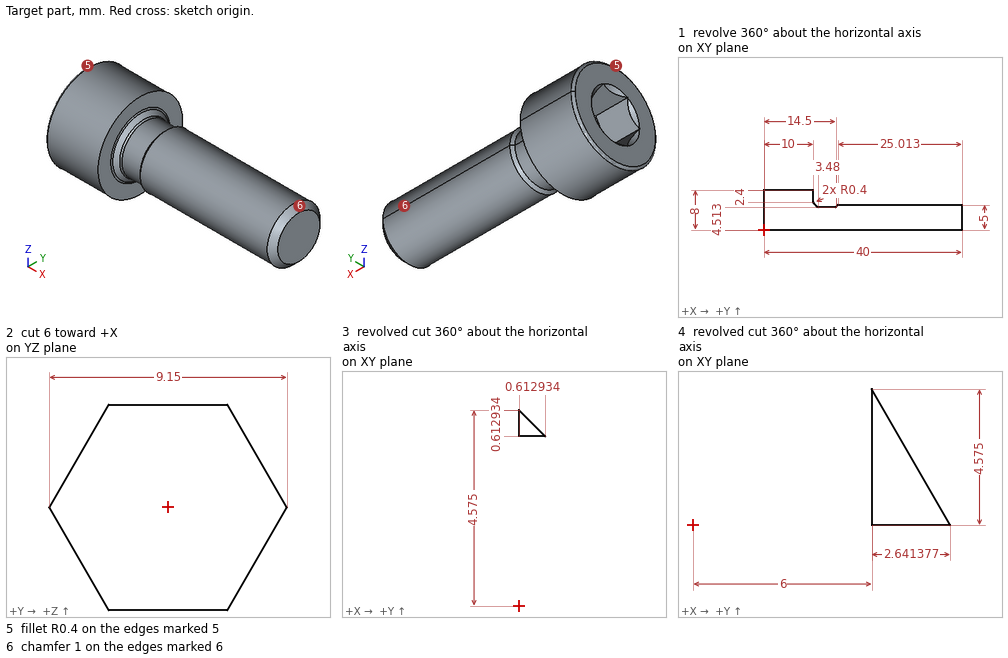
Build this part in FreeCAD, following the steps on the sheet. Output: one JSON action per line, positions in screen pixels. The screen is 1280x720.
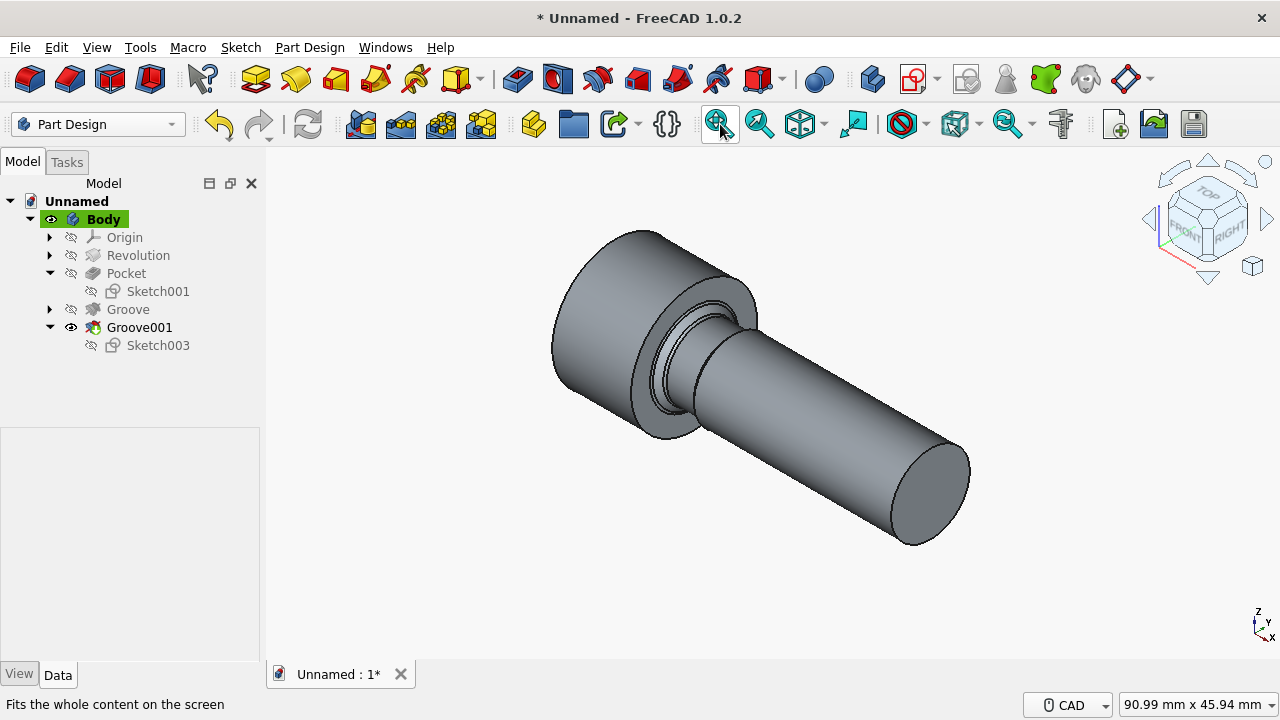
{"action": "key", "text": "2"}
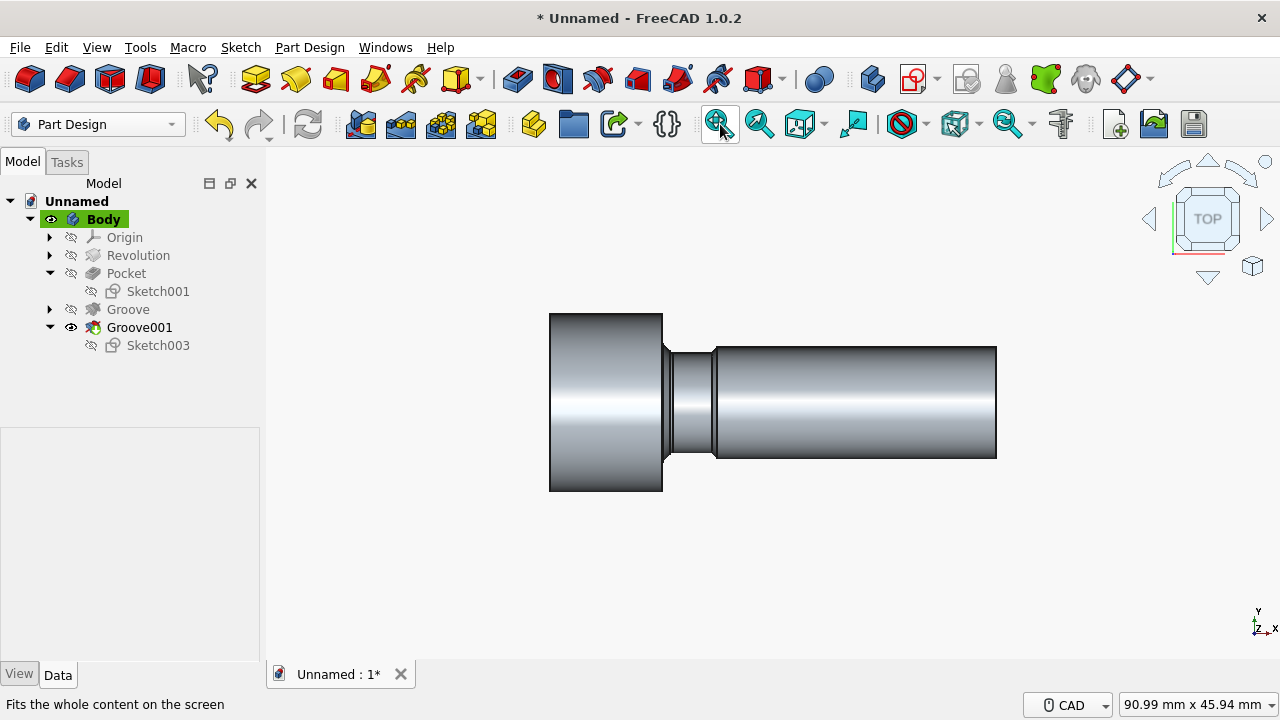
{"action": "left_click", "coordinate": [720, 124]}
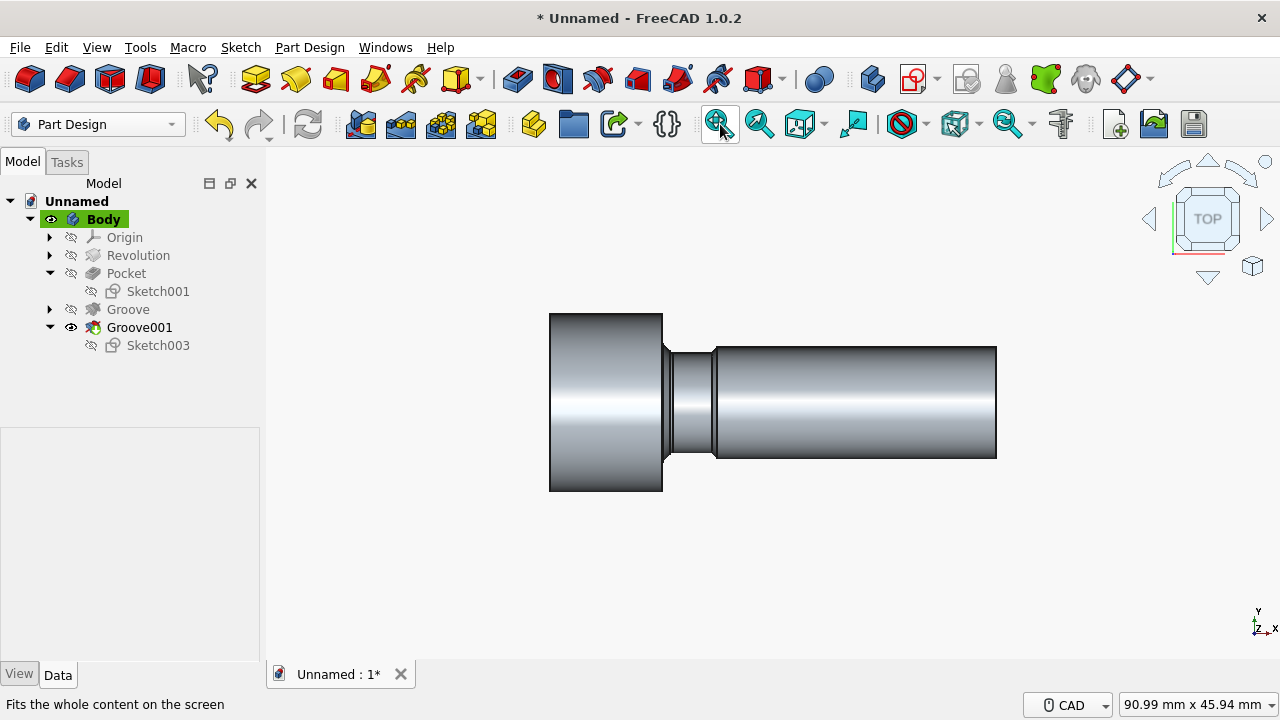
{"action": "left_click", "coordinate": [550, 474]}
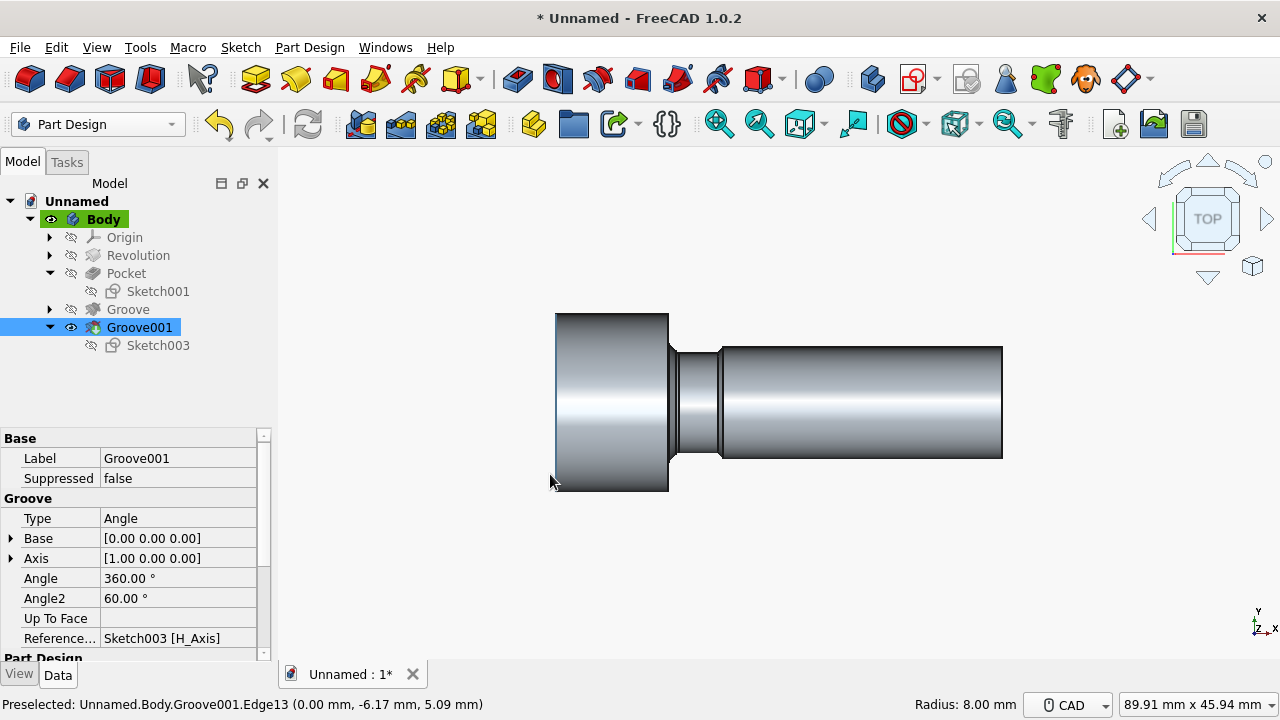
{"action": "left_click", "coordinate": [30, 80]}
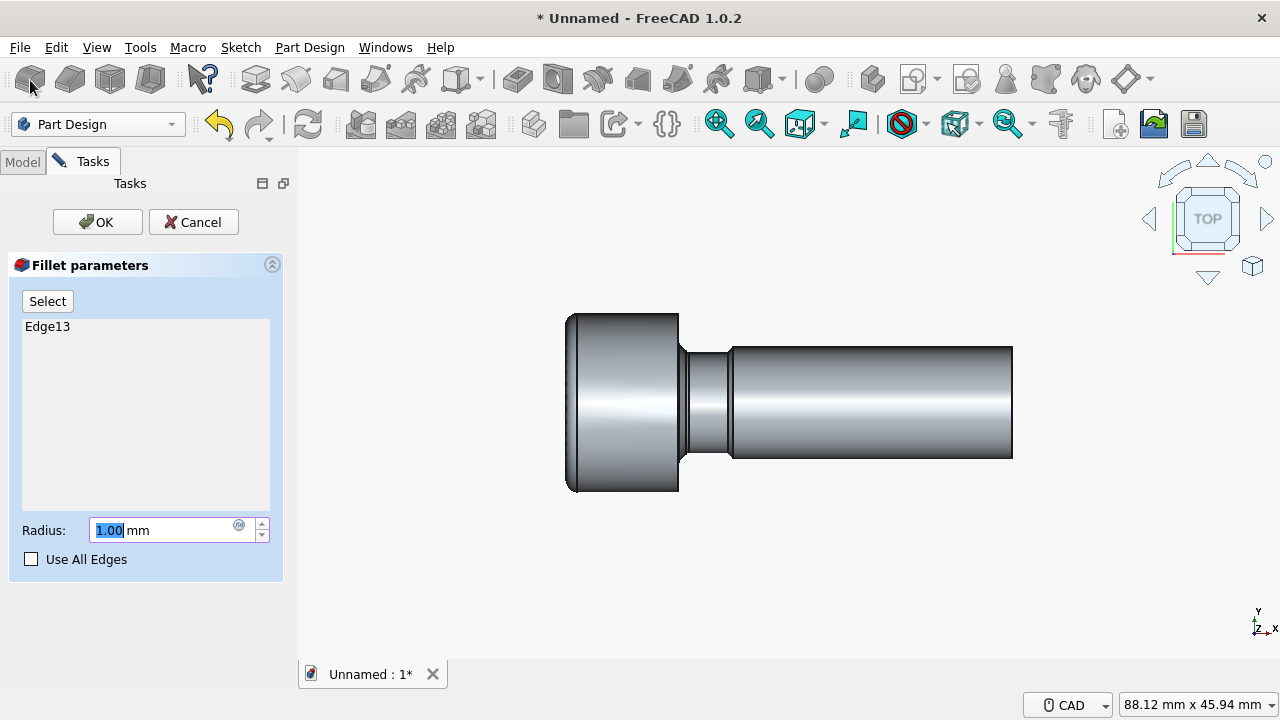
{"action": "type", "text": "0.4"}
{"action": "key", "text": "Tab"}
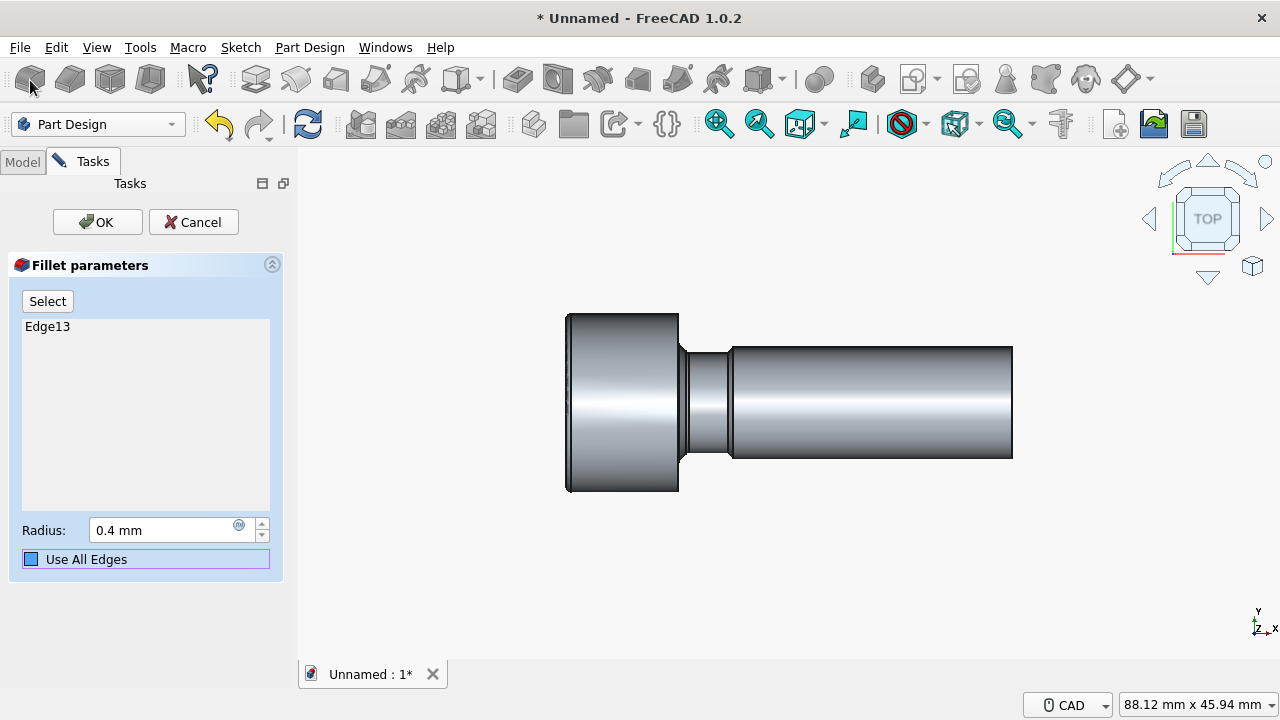
{"action": "left_click", "coordinate": [98, 222]}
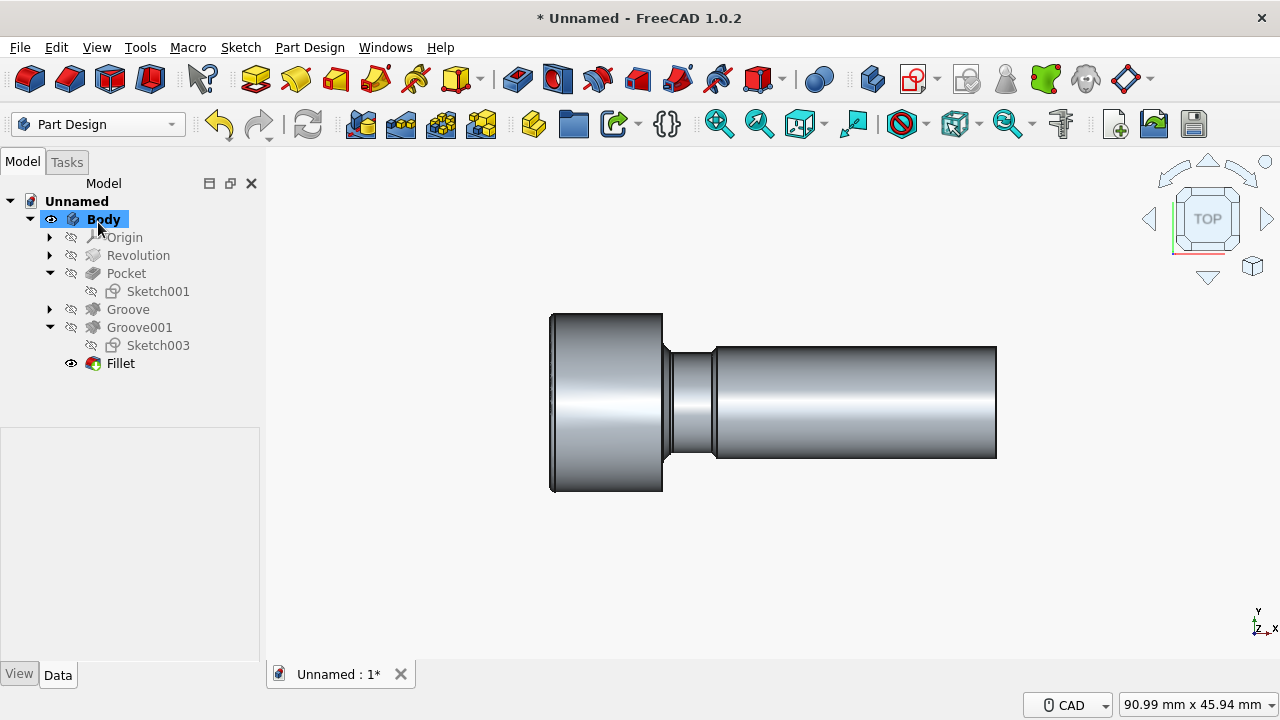
{"action": "left_click", "coordinate": [720, 124]}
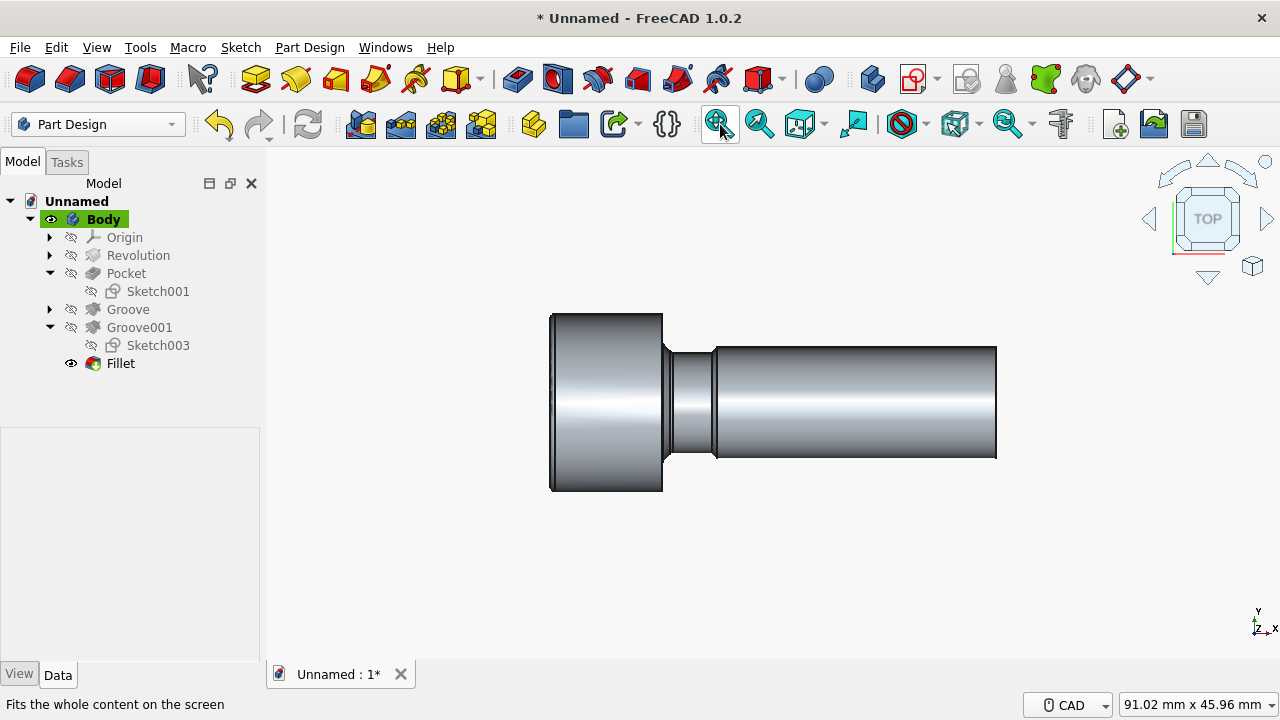
{"action": "left_click", "coordinate": [996, 447]}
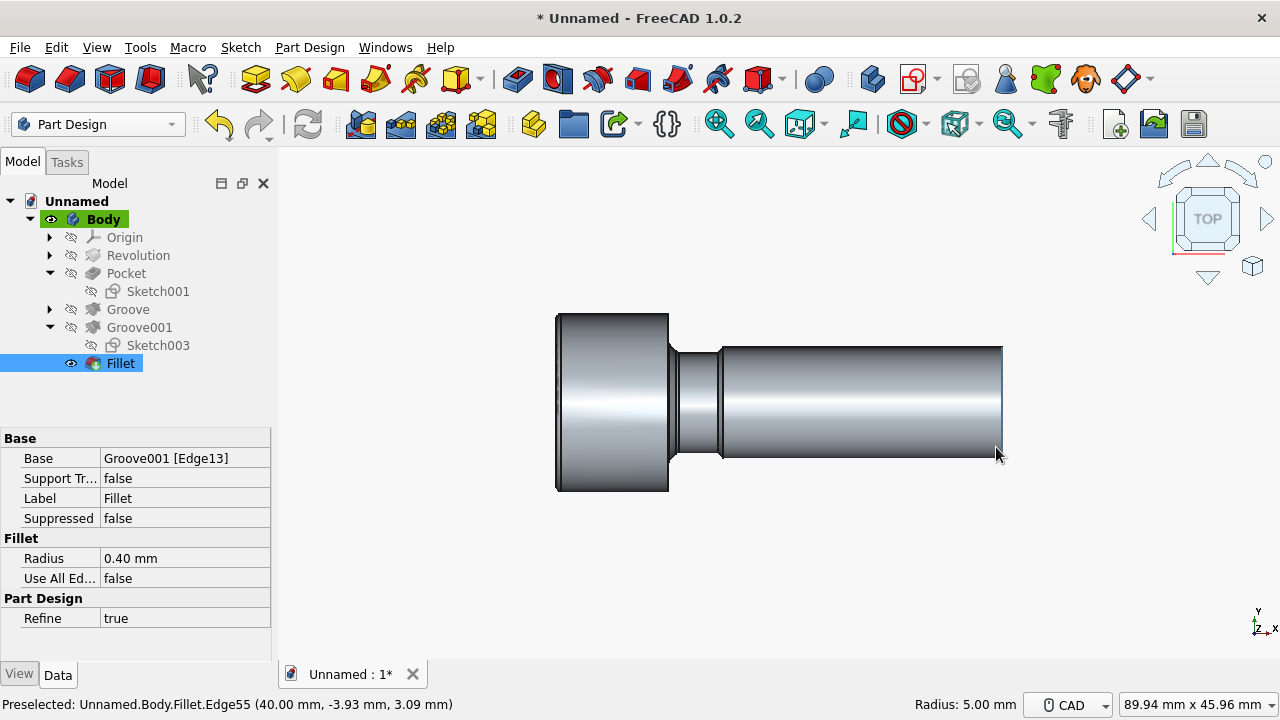
{"action": "left_click", "coordinate": [70, 80]}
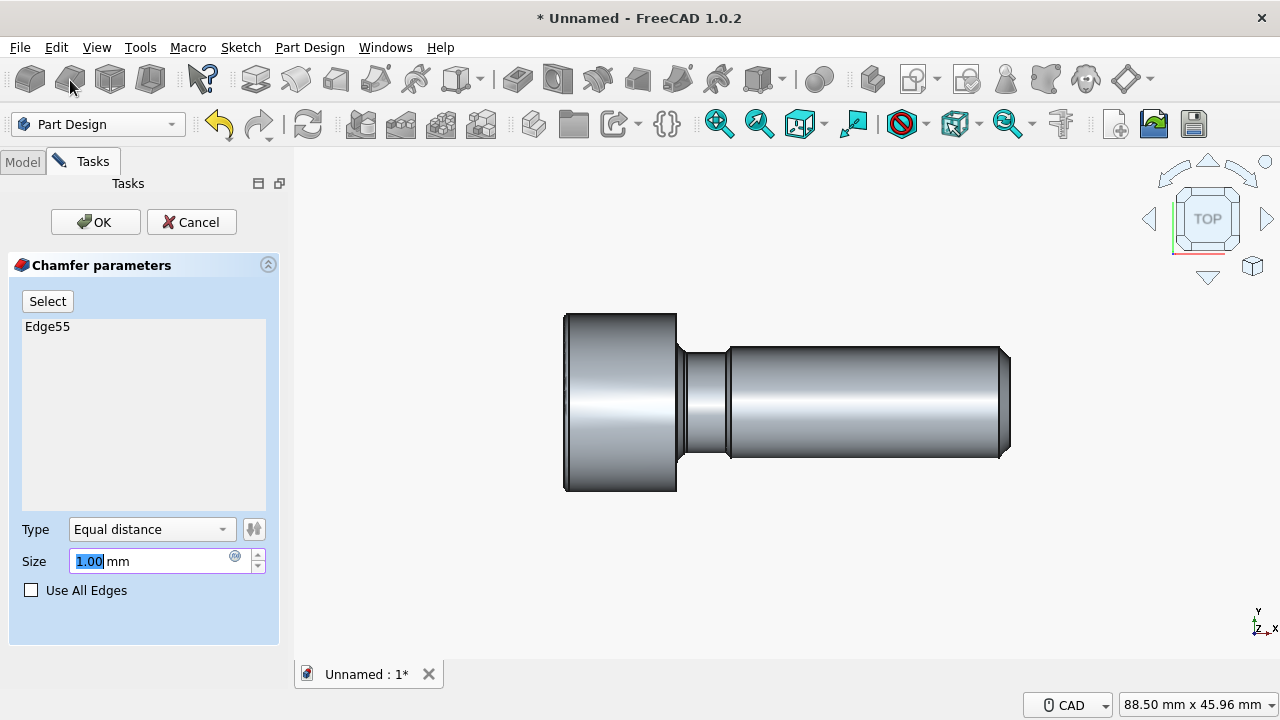
{"action": "type", "text": "1"}
{"action": "key", "text": "Tab"}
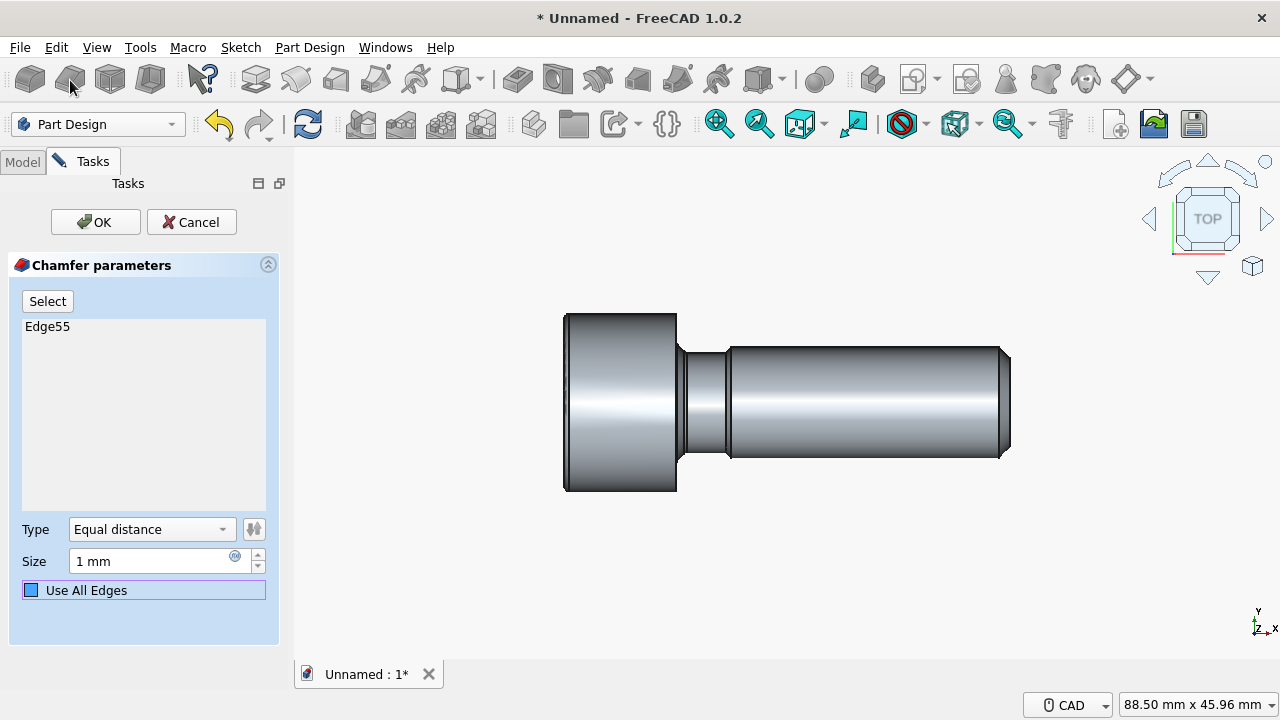
{"action": "left_click", "coordinate": [96, 222]}